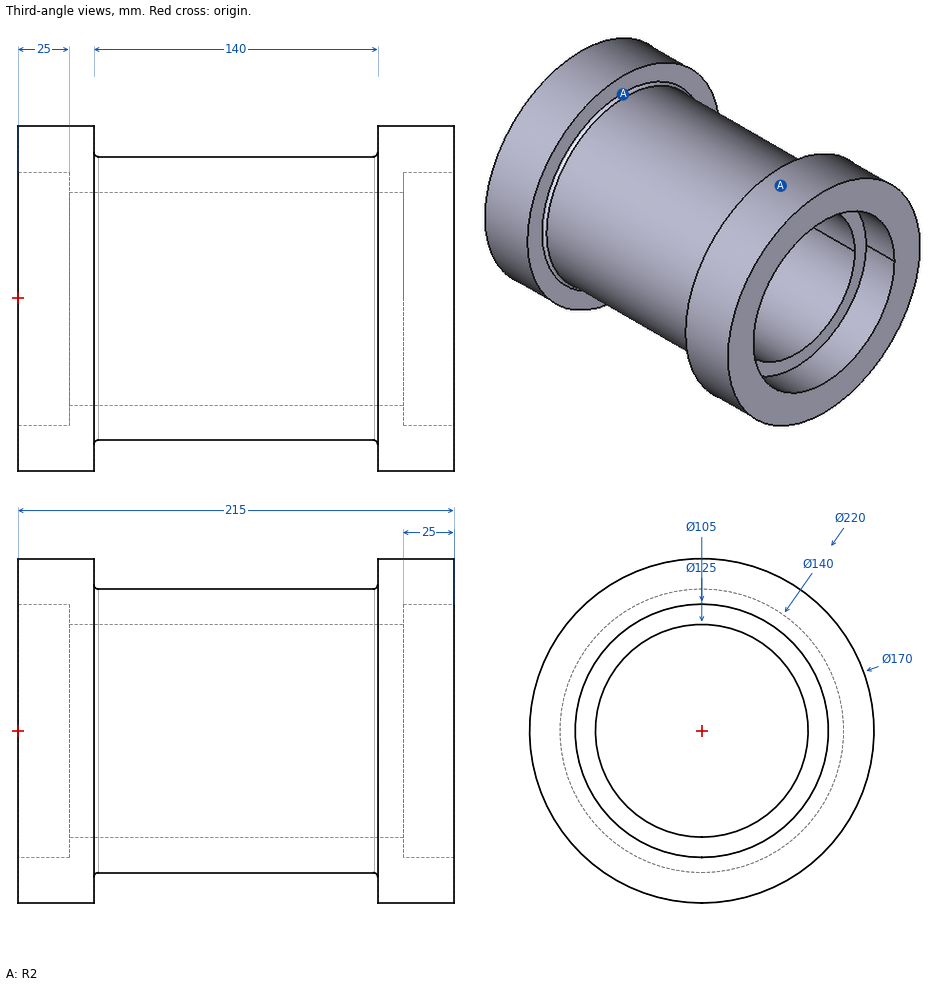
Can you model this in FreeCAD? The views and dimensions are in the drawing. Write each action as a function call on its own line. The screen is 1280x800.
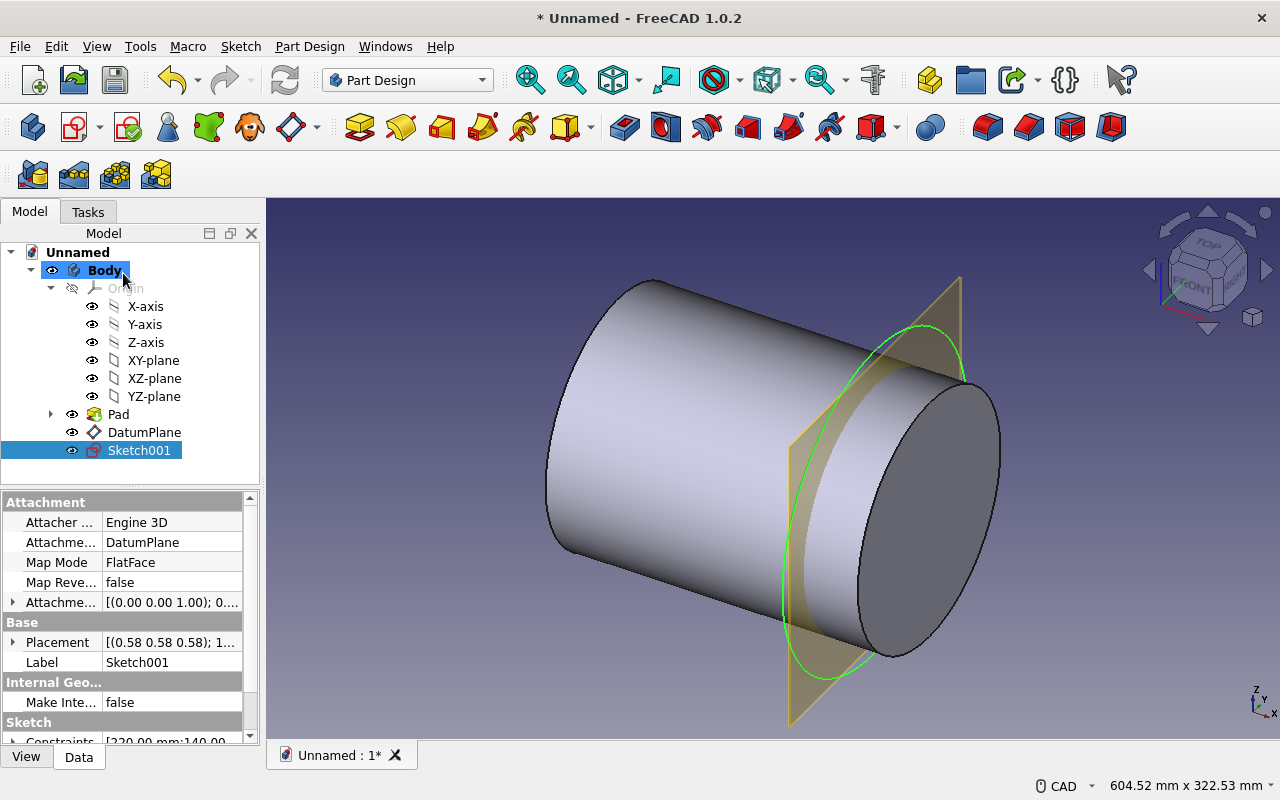
click(625, 128)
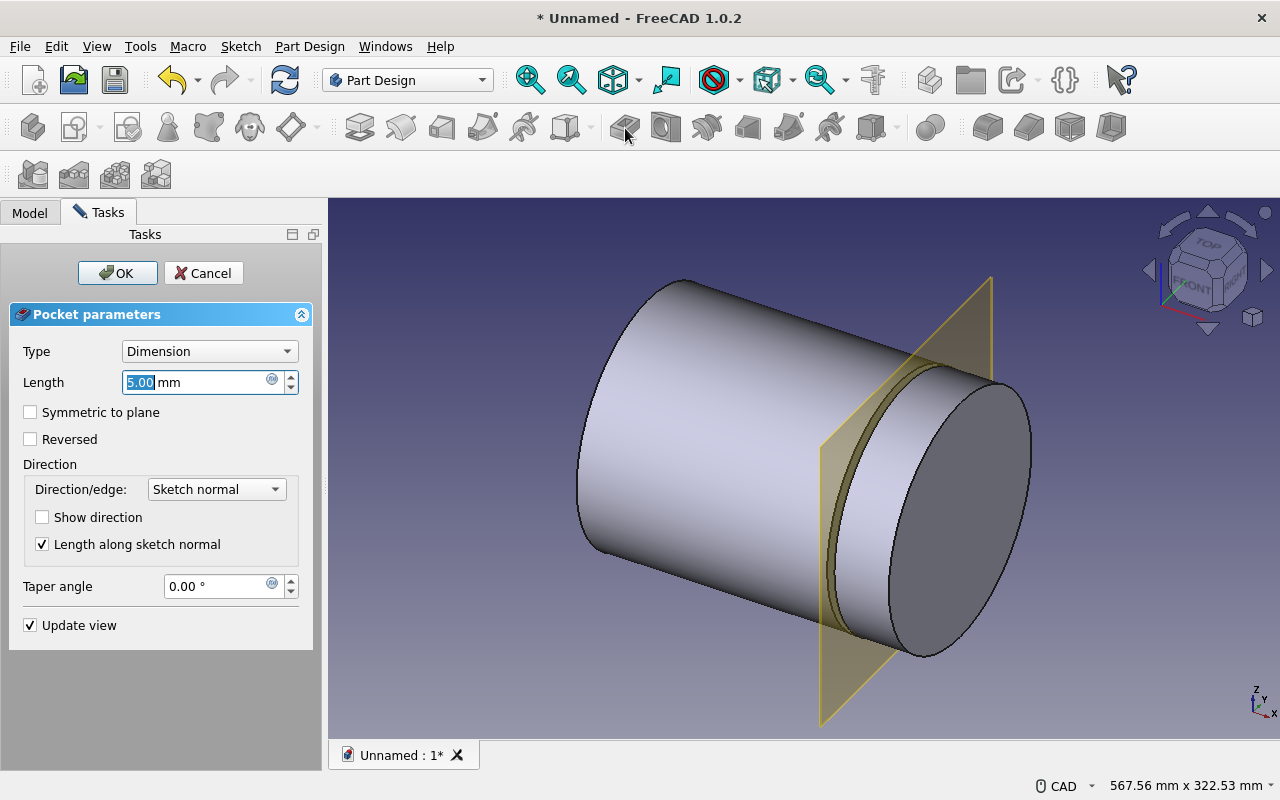
text(140)
key(Tab)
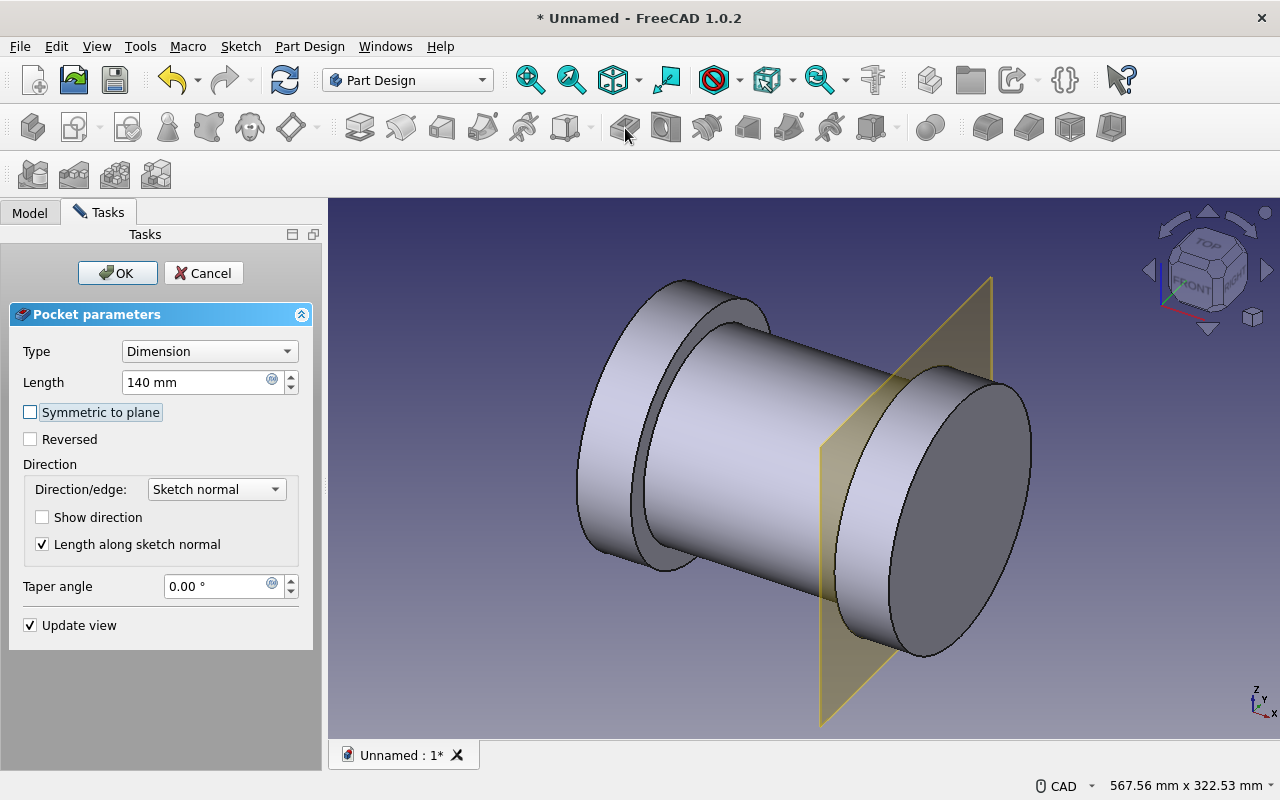
click(118, 273)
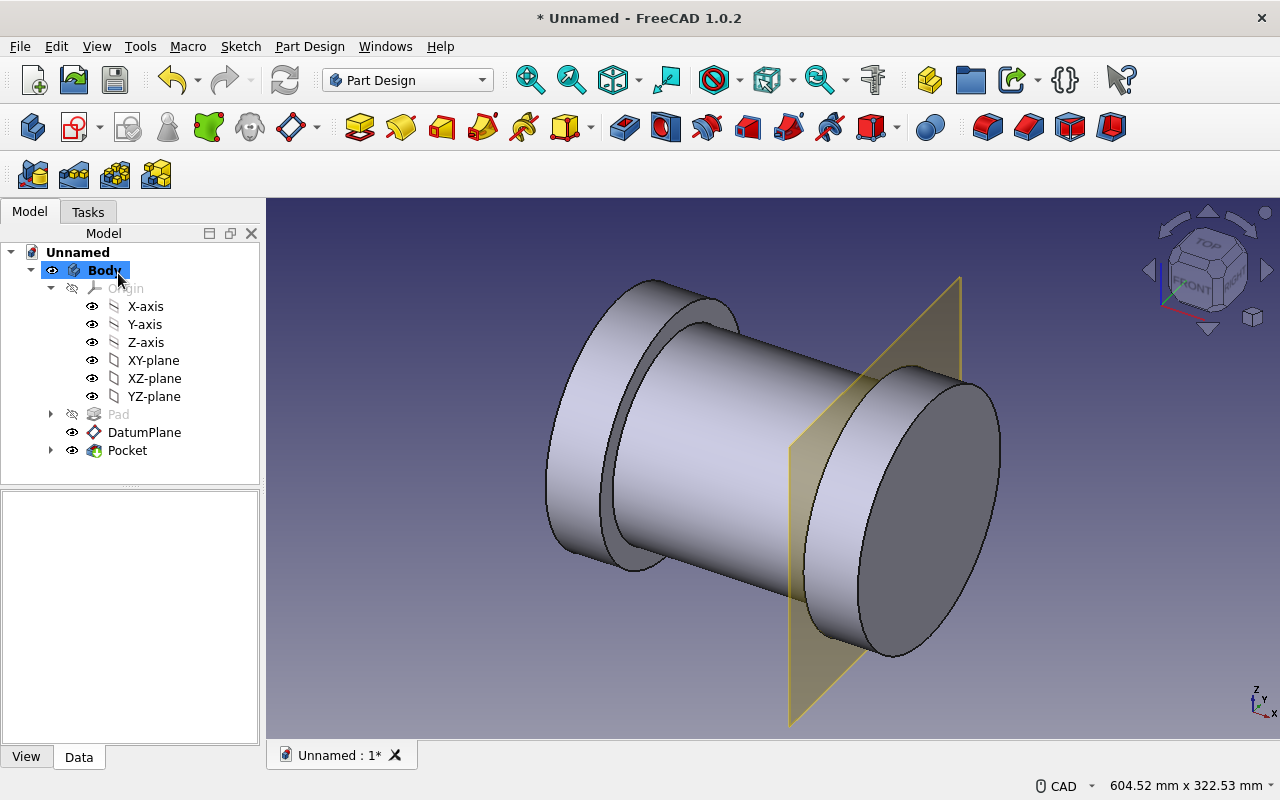
click(117, 432)
key(space)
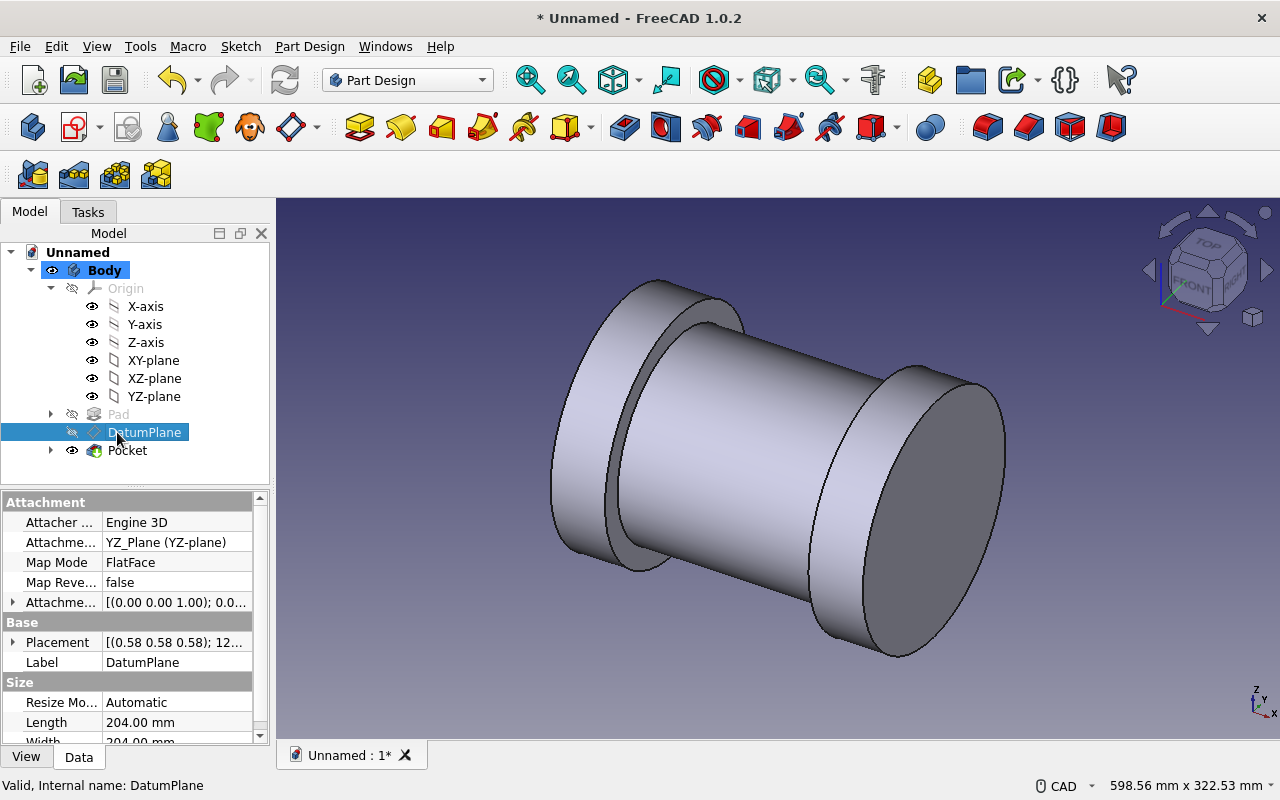
key(0)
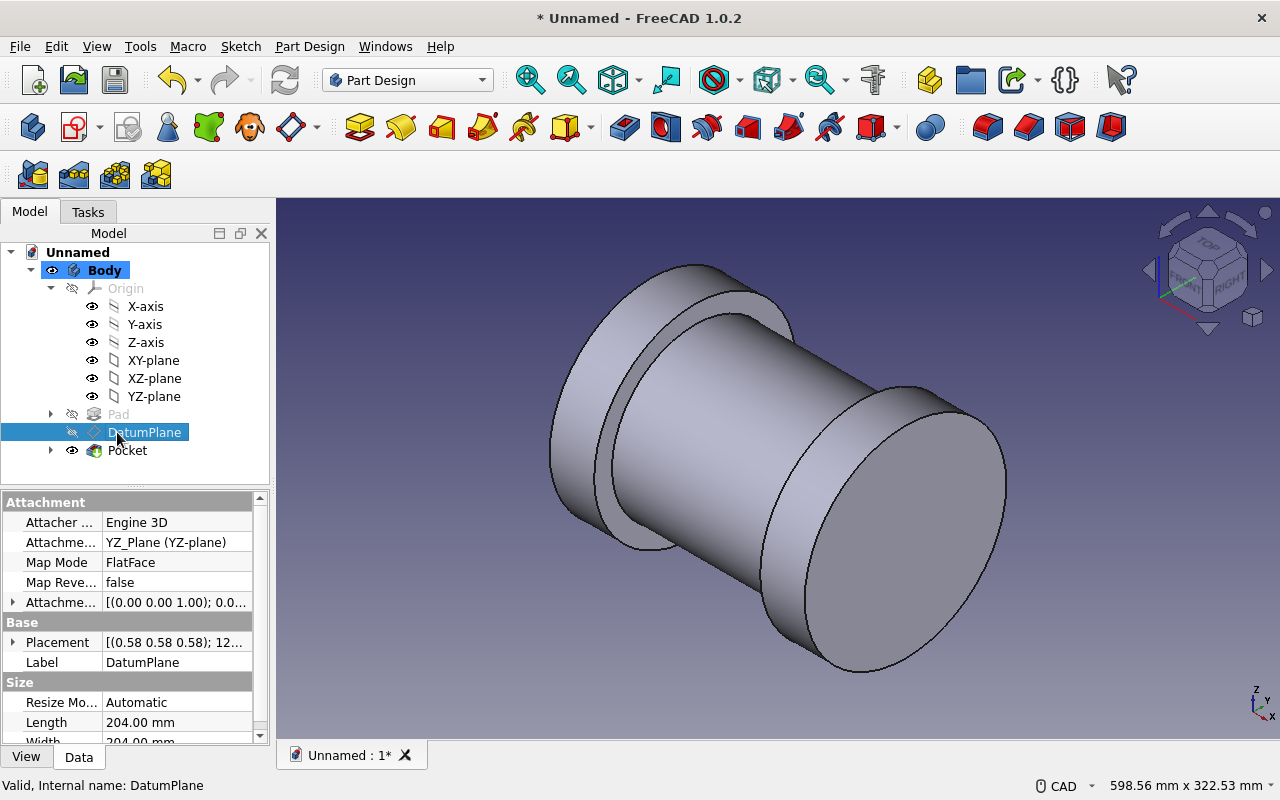
key(2)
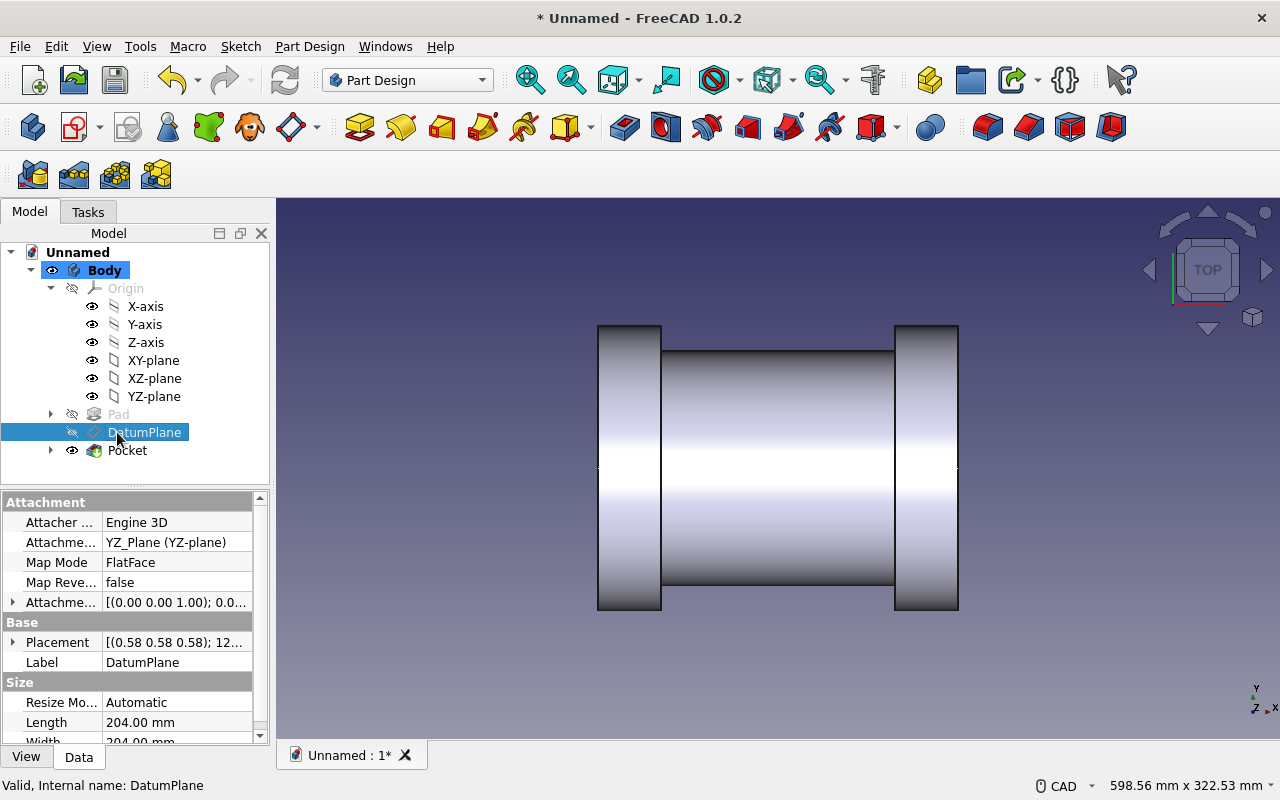
key(1)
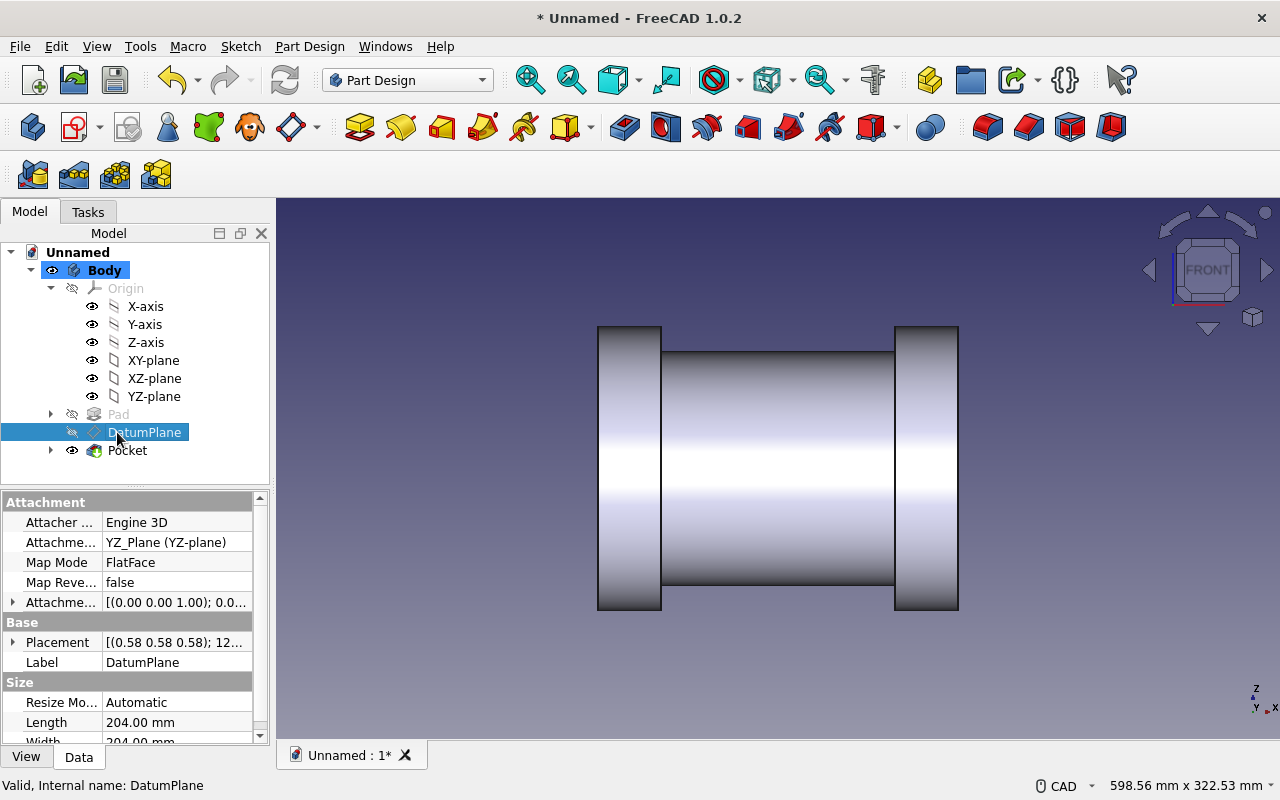
key(3)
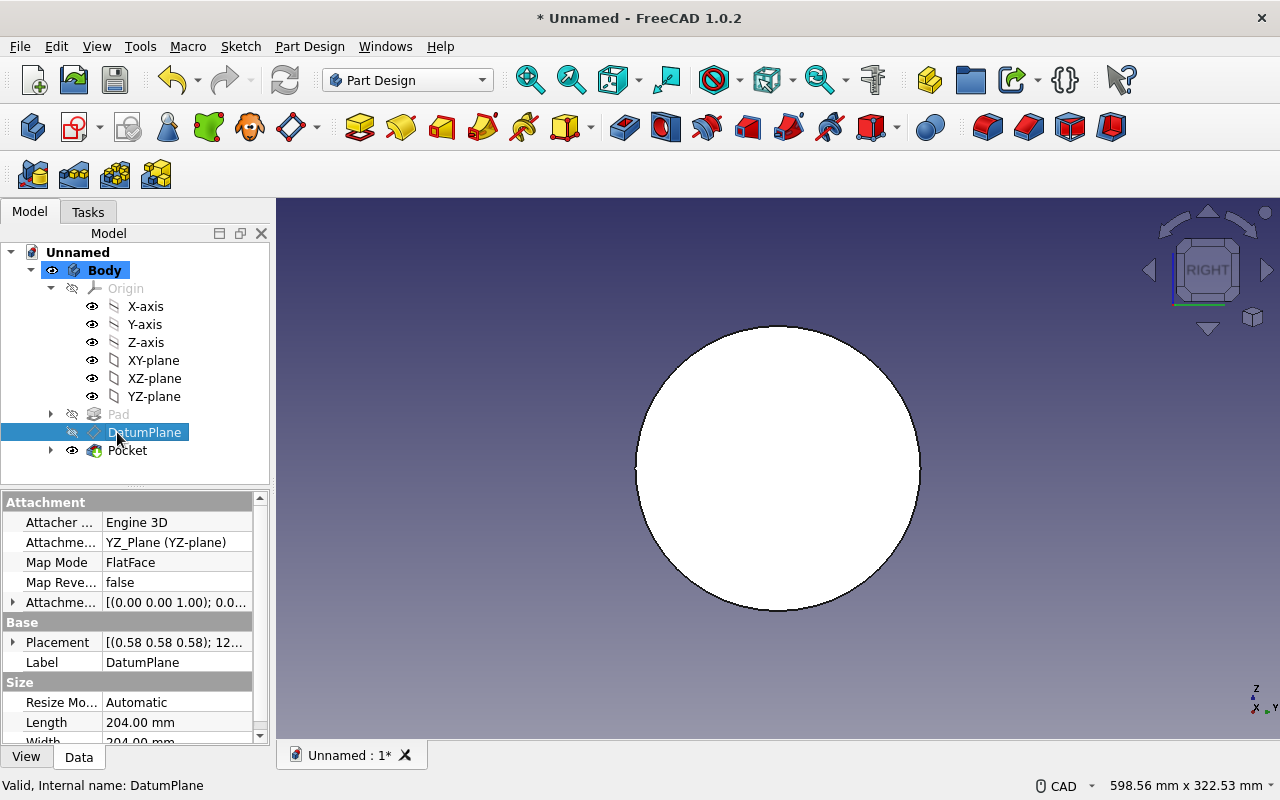
key(5)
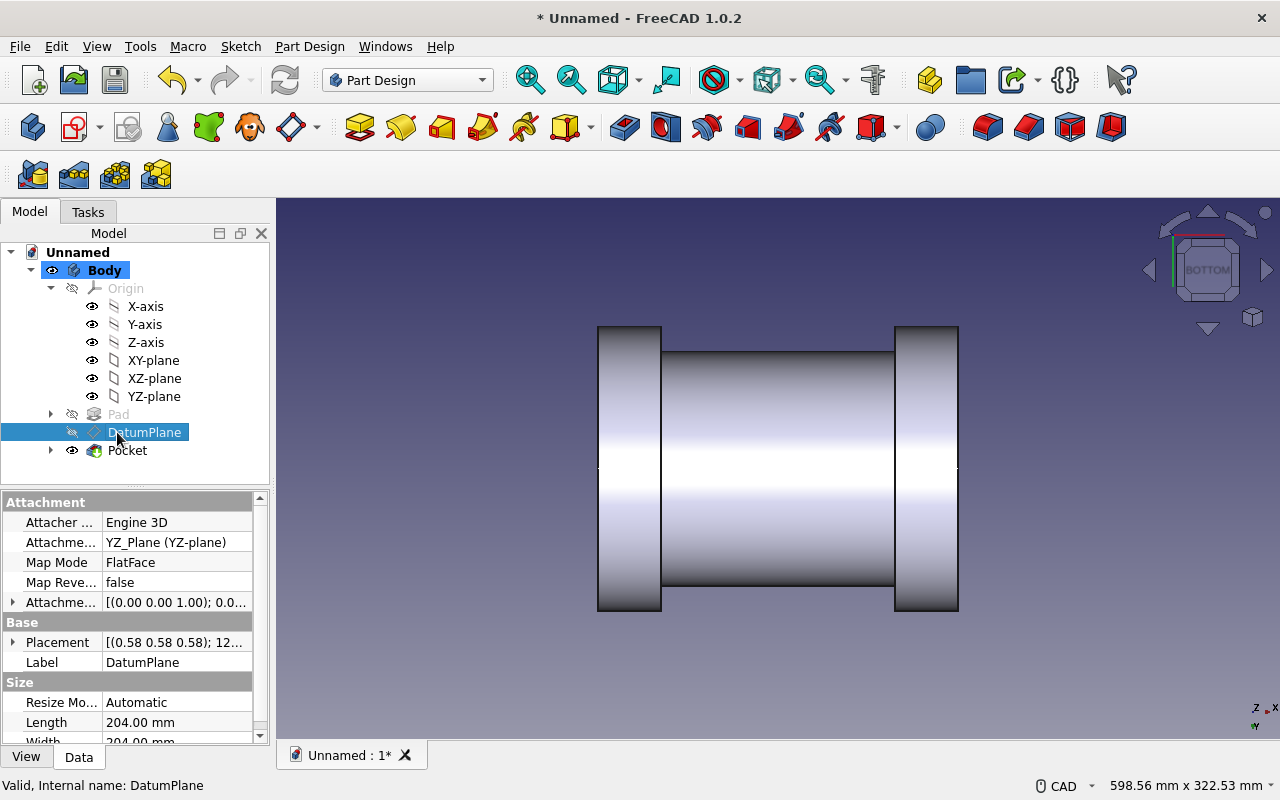
key(4)